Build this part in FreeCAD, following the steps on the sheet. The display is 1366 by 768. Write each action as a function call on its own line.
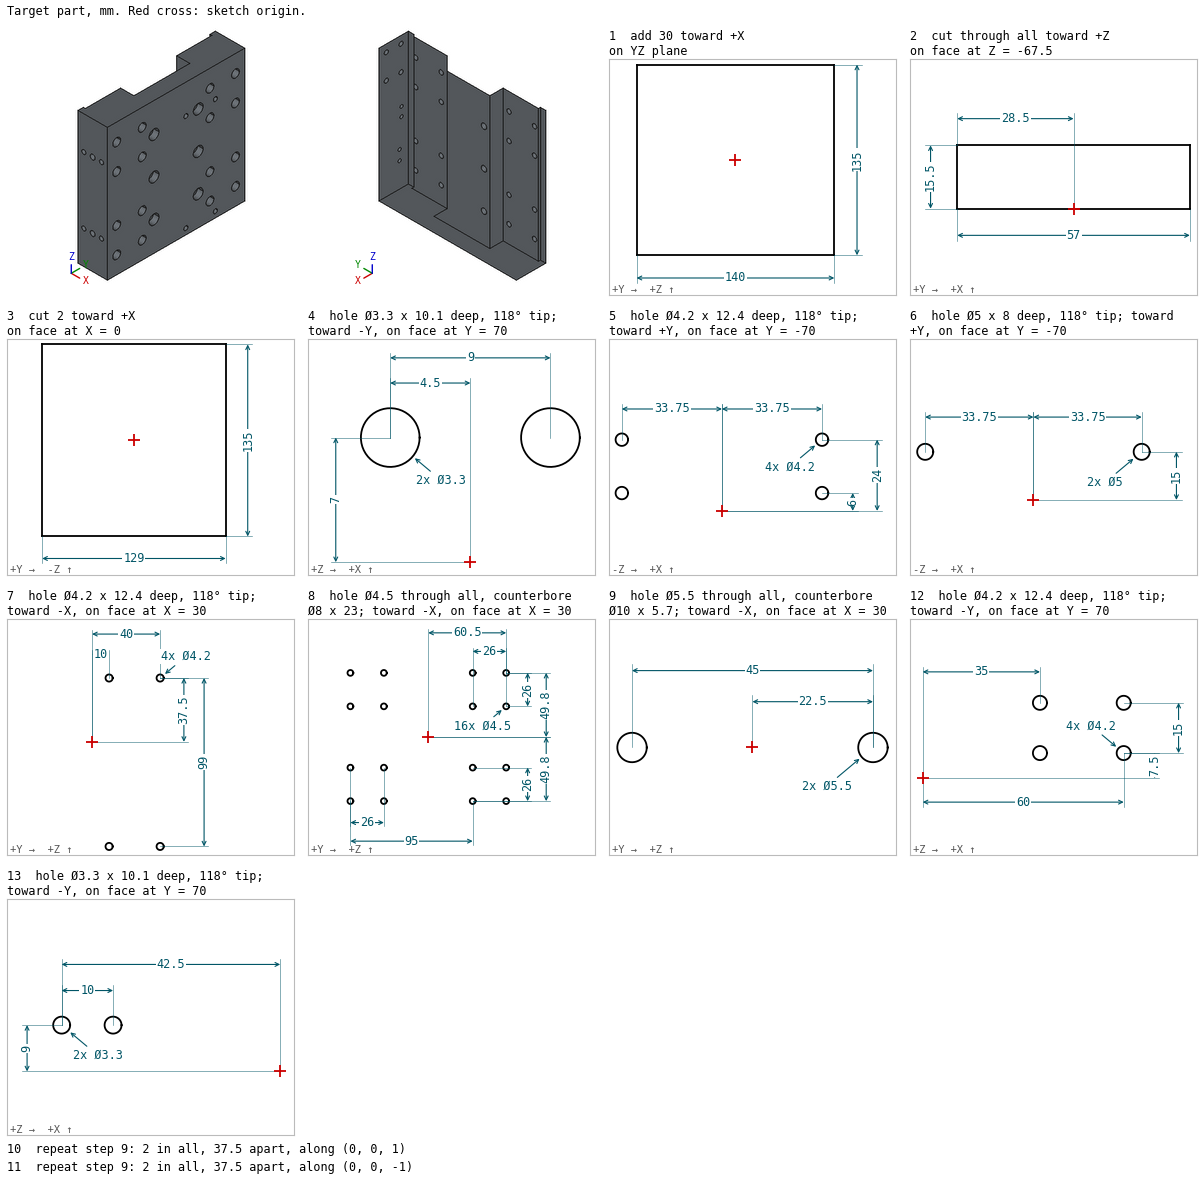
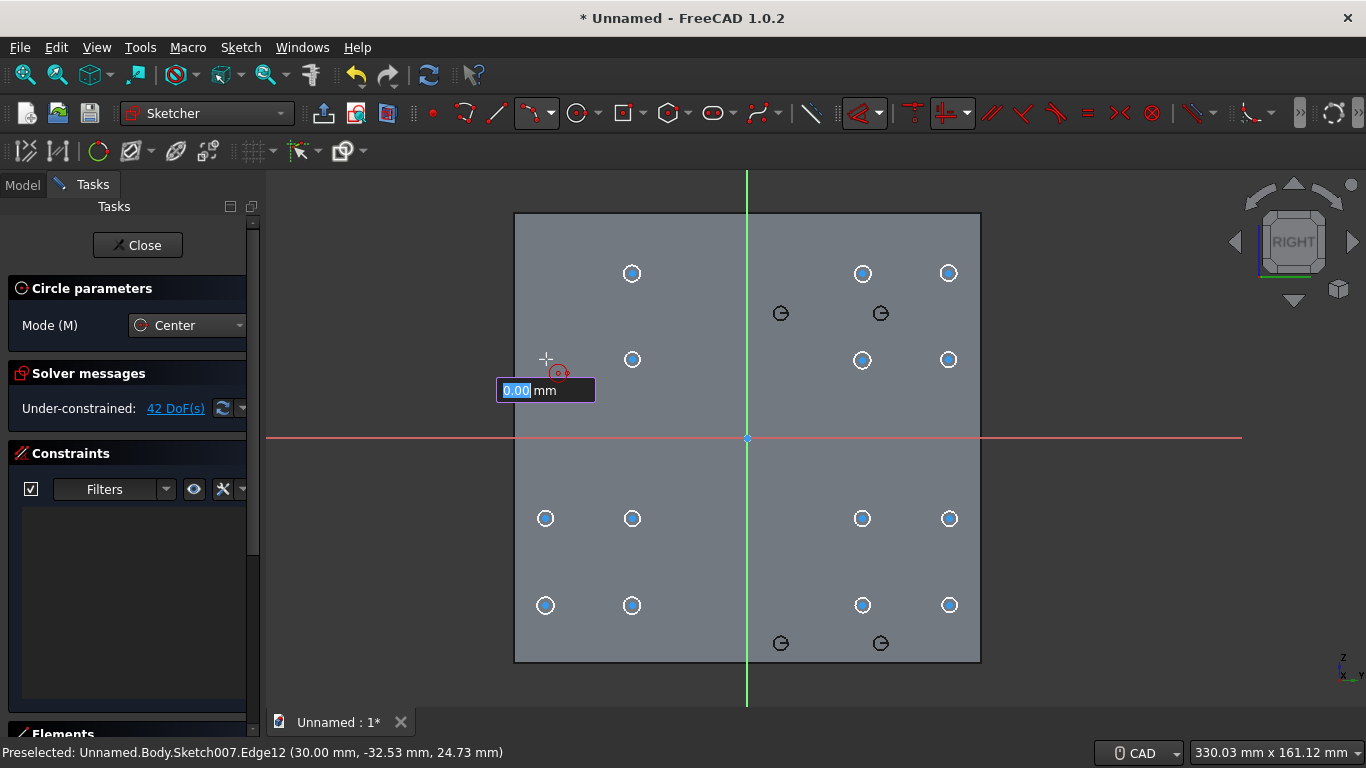
scroll(551, 354, up, 4)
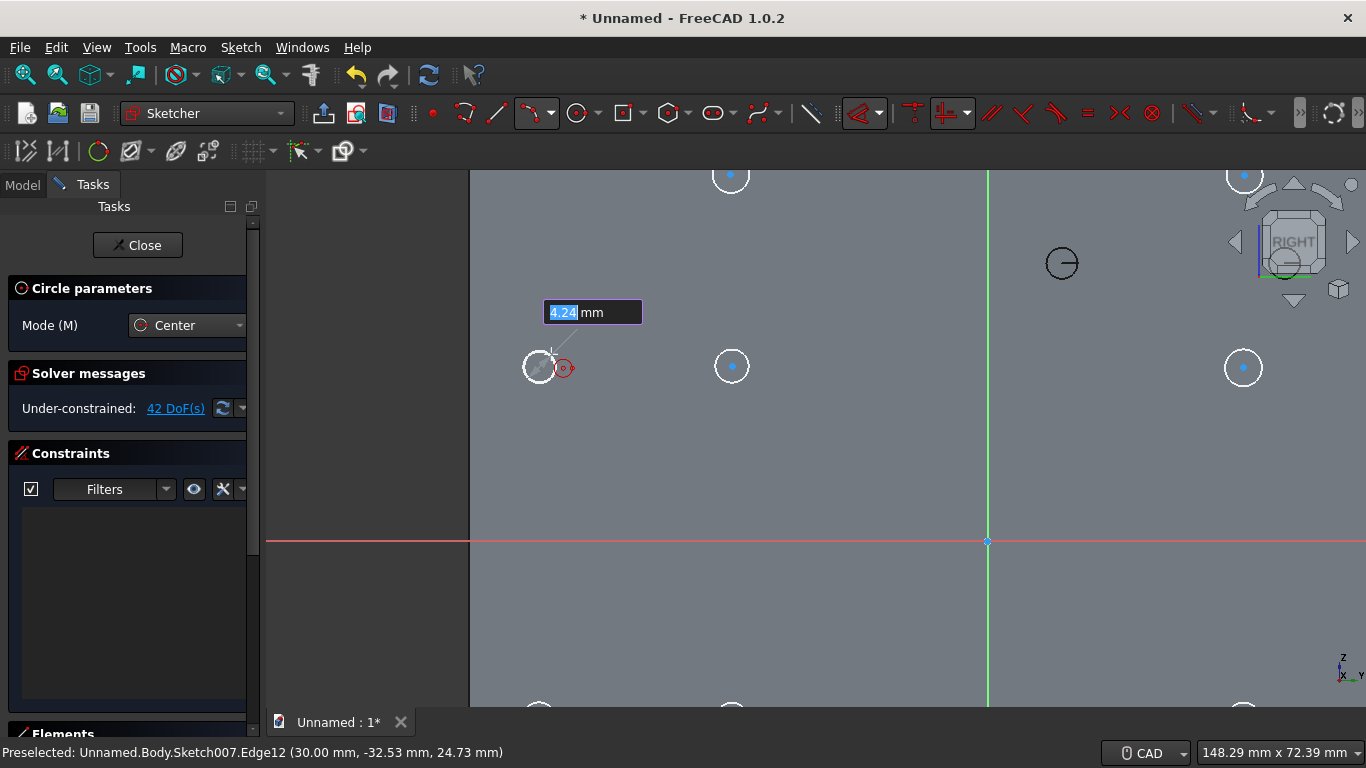
click(551, 353)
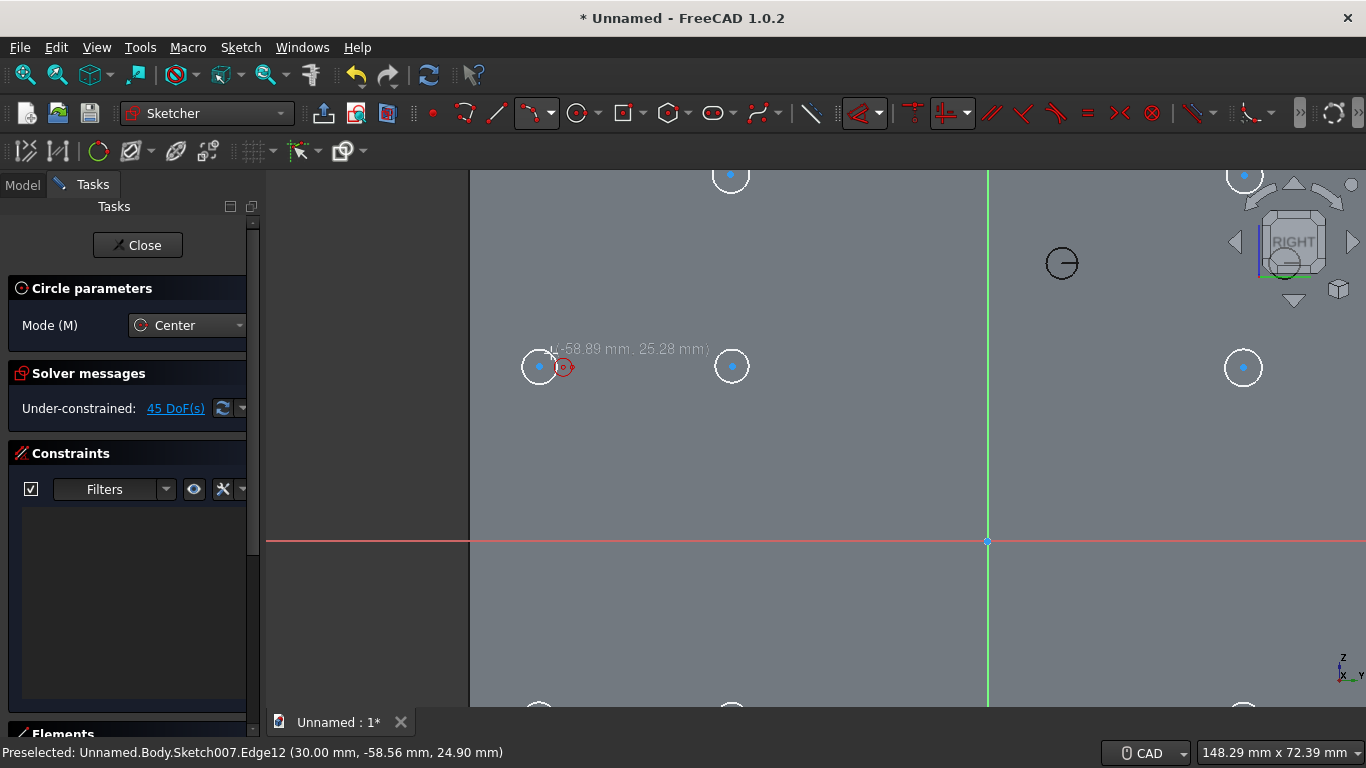
scroll(551, 354, down, 4)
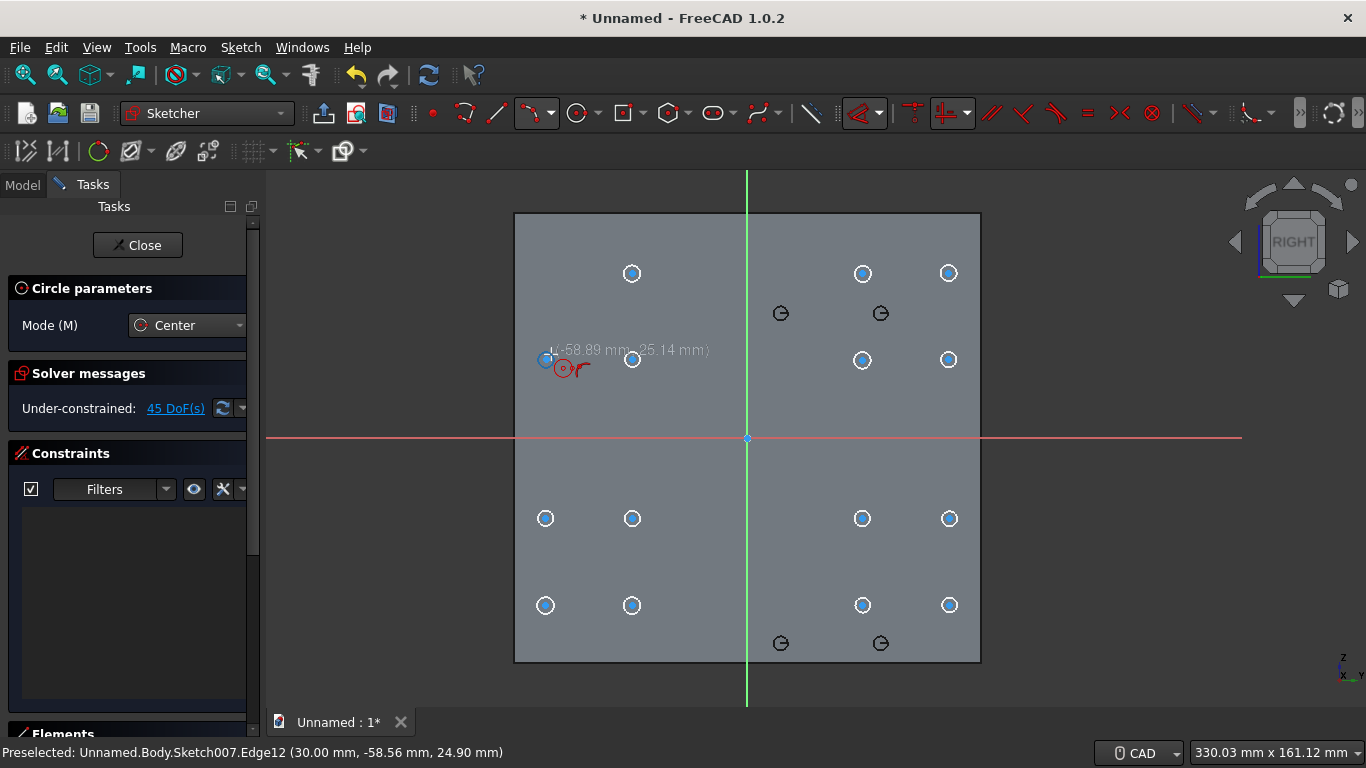
scroll(546, 272, up, 6)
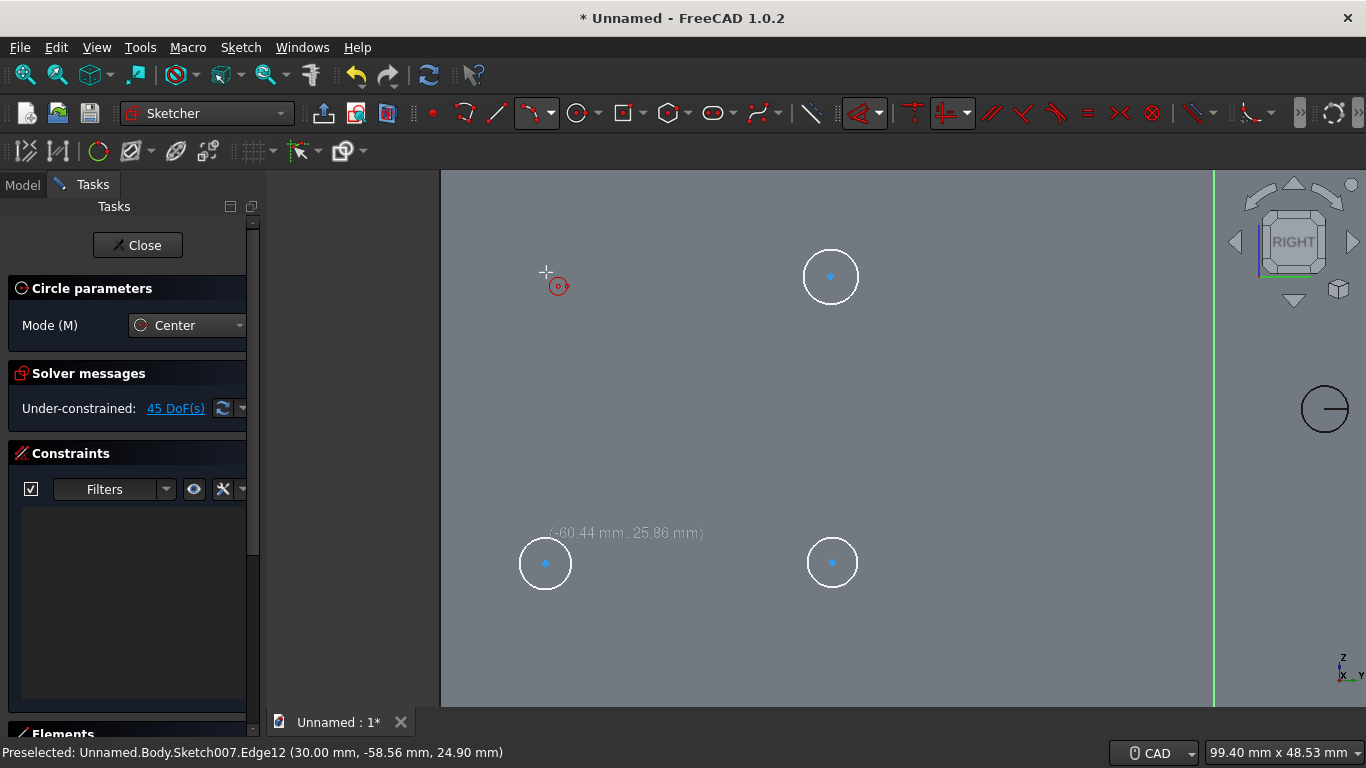
scroll(546, 272, down, 6)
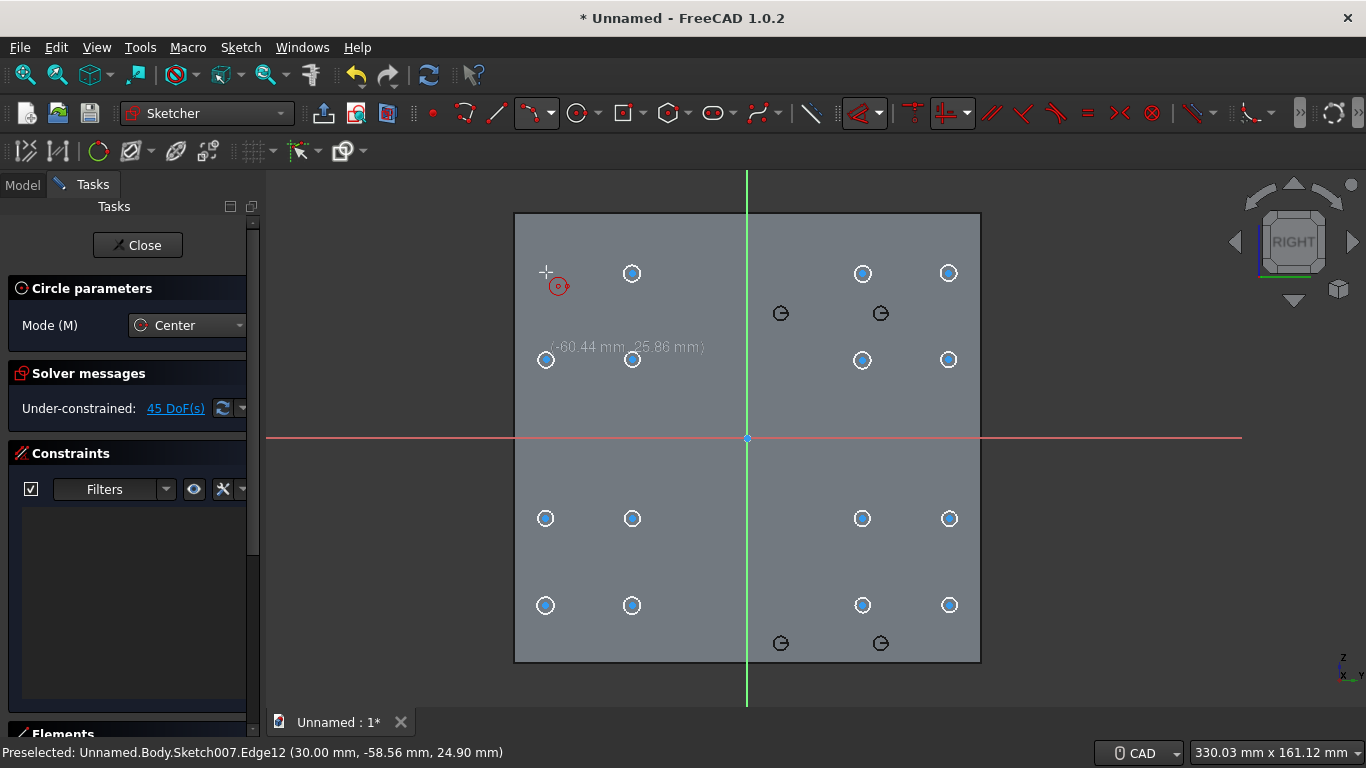
click(546, 272)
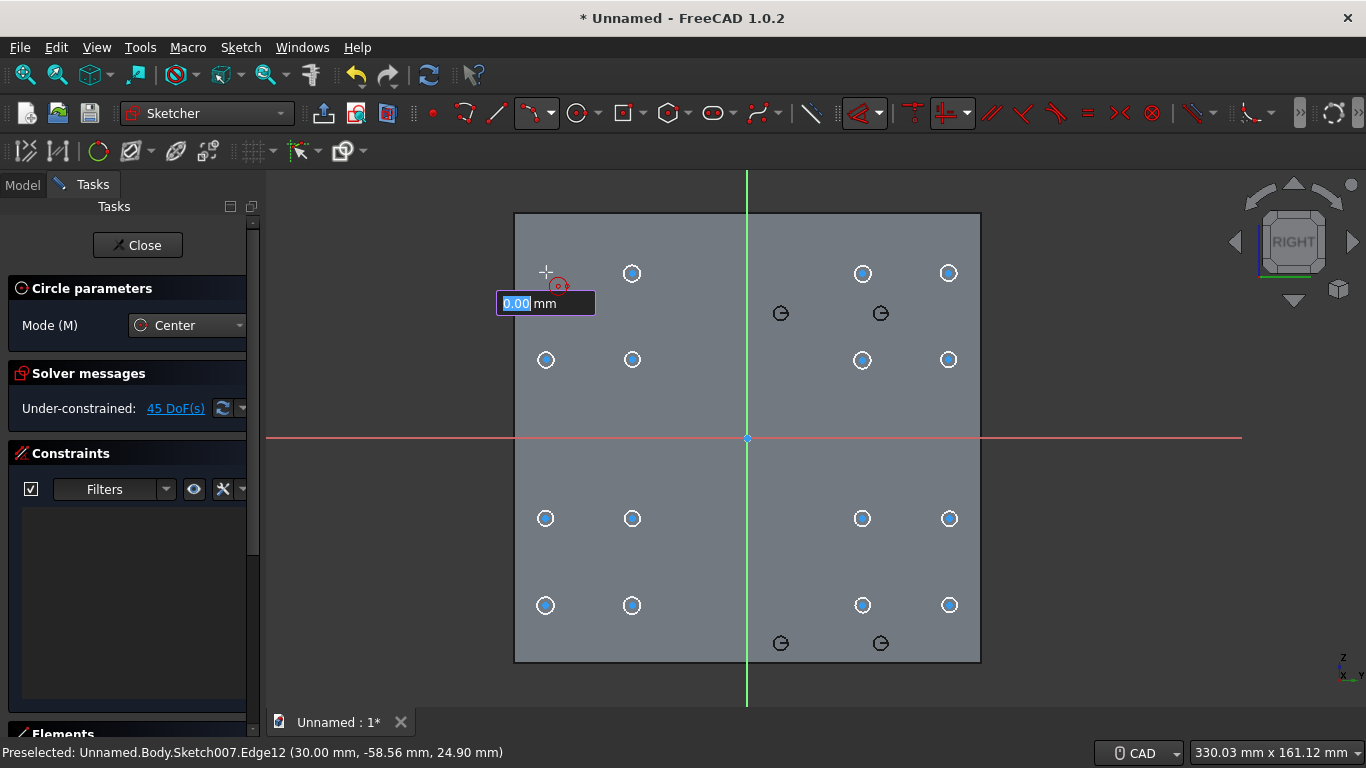
scroll(551, 267, up, 4)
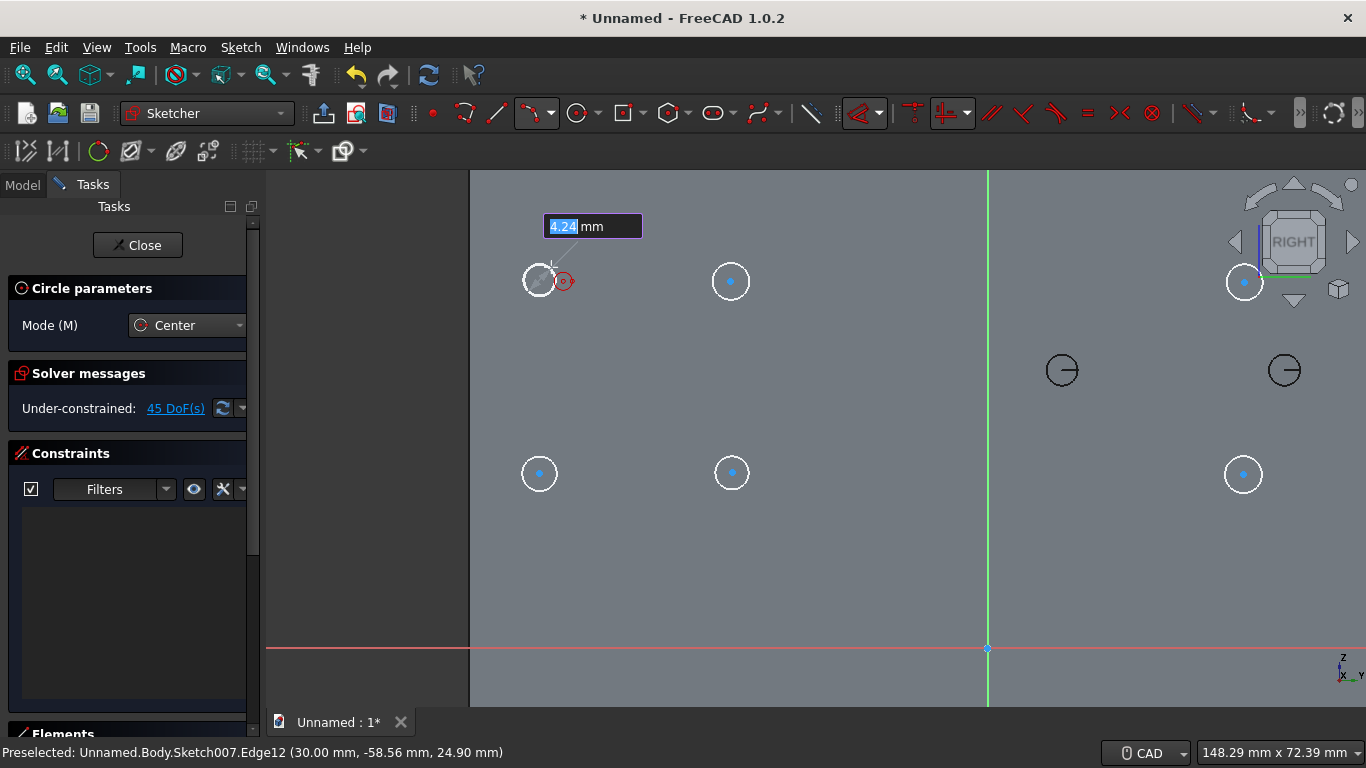
click(551, 267)
key(Escape)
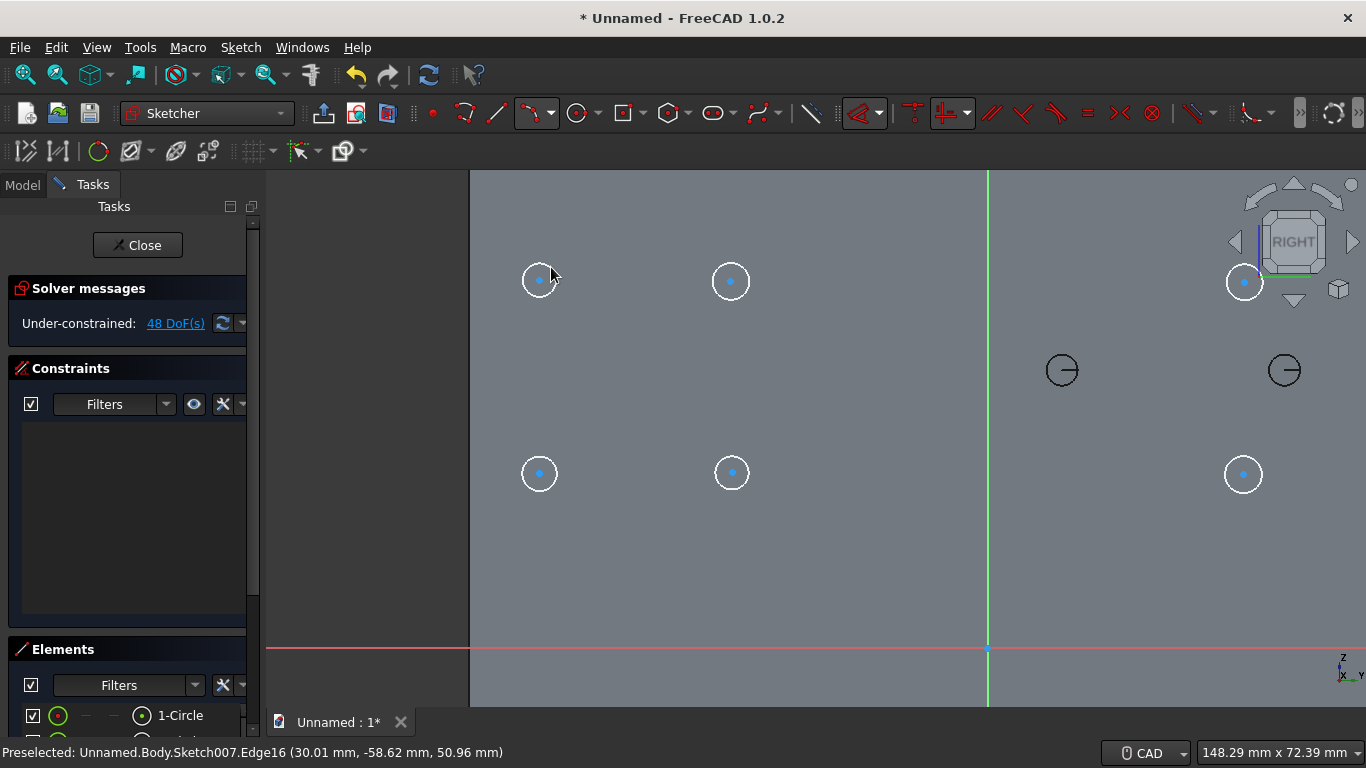
scroll(551, 267, down, 4)